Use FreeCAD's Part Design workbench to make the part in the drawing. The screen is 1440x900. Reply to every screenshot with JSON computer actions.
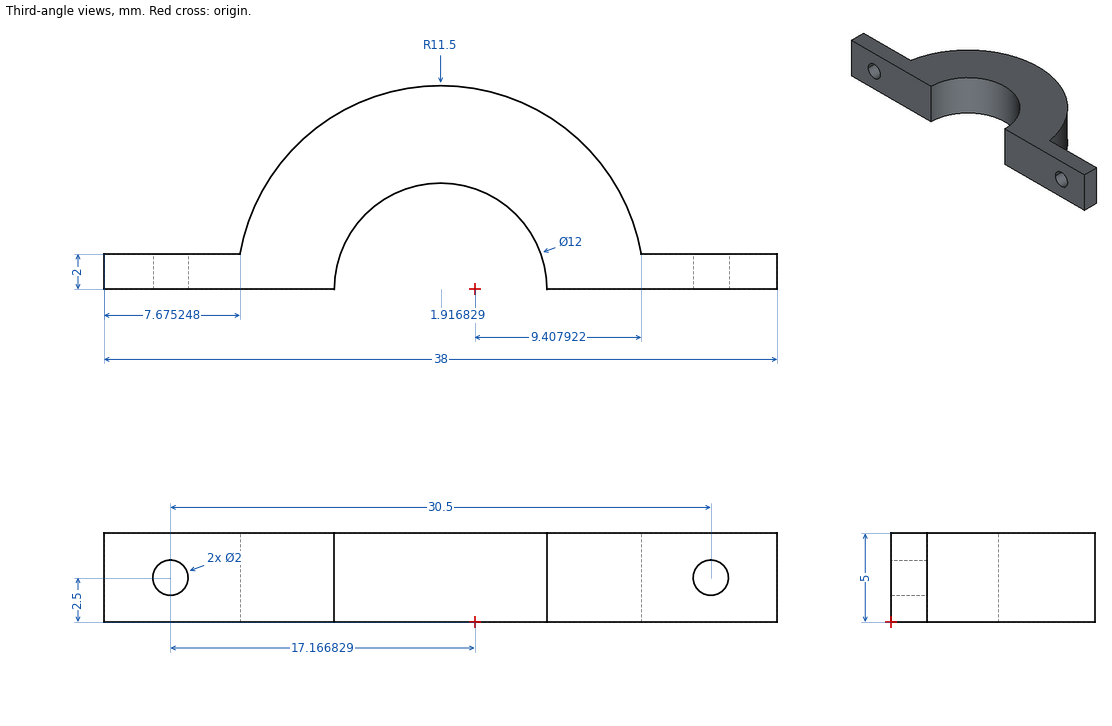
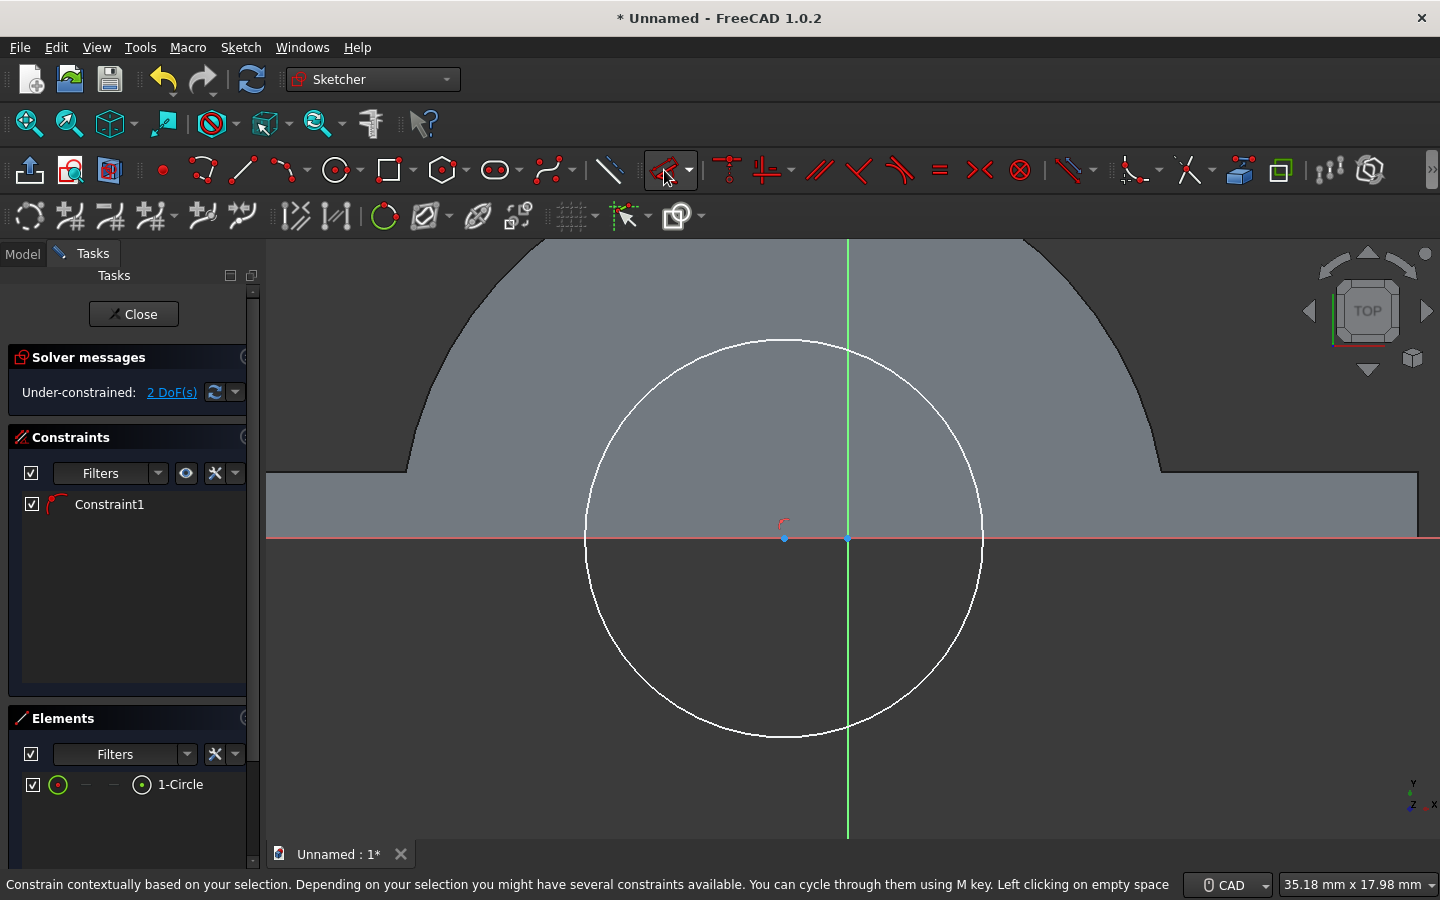
{"action": "left_click", "coordinate": [924, 397]}
{"action": "left_click", "coordinate": [947, 374]}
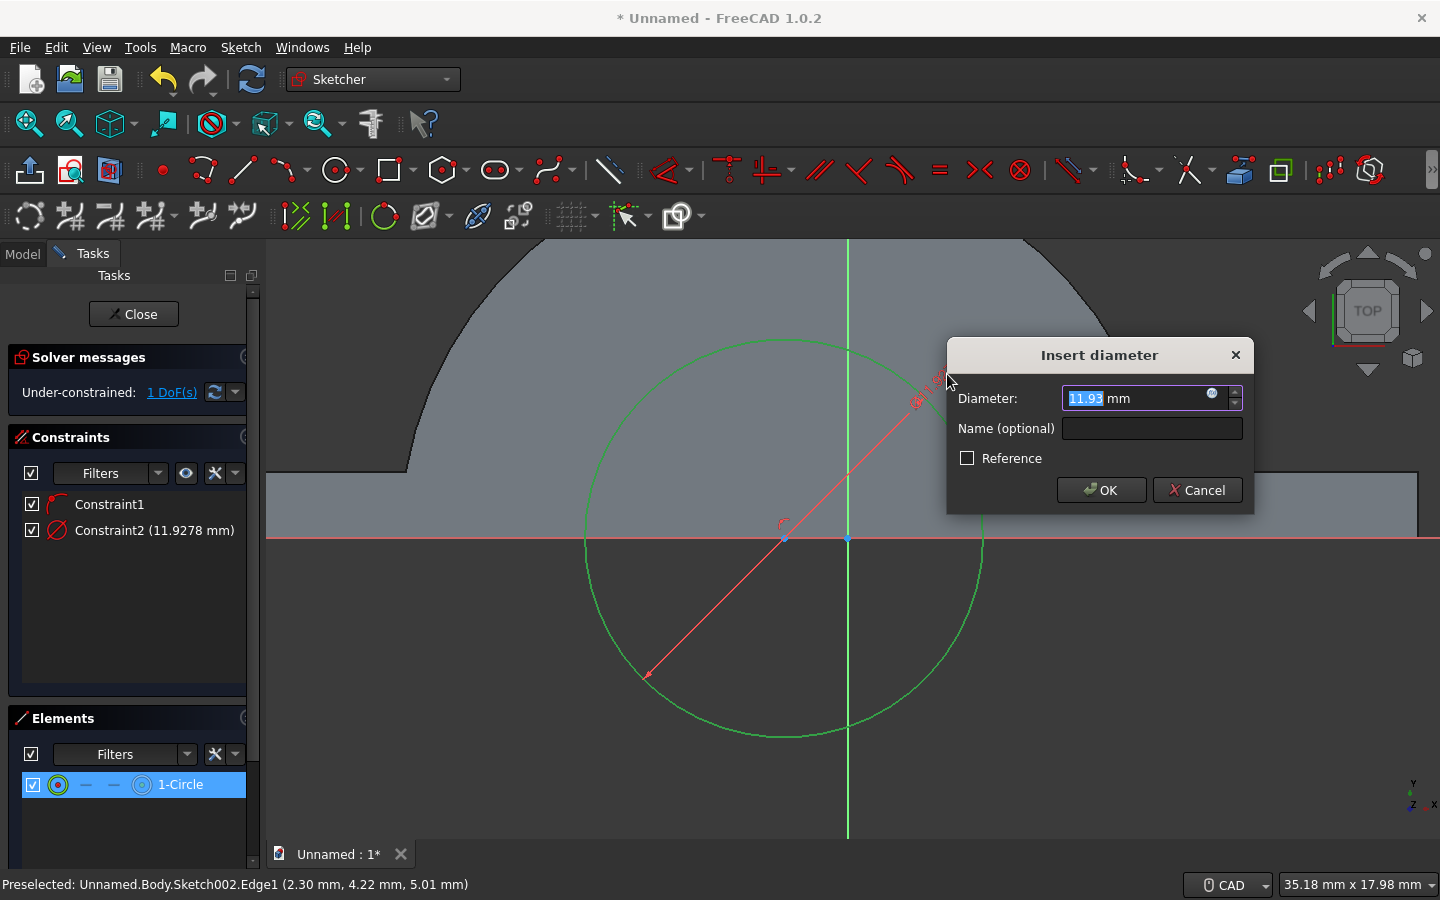
{"action": "type", "text": "12"}
{"action": "key", "text": "Return"}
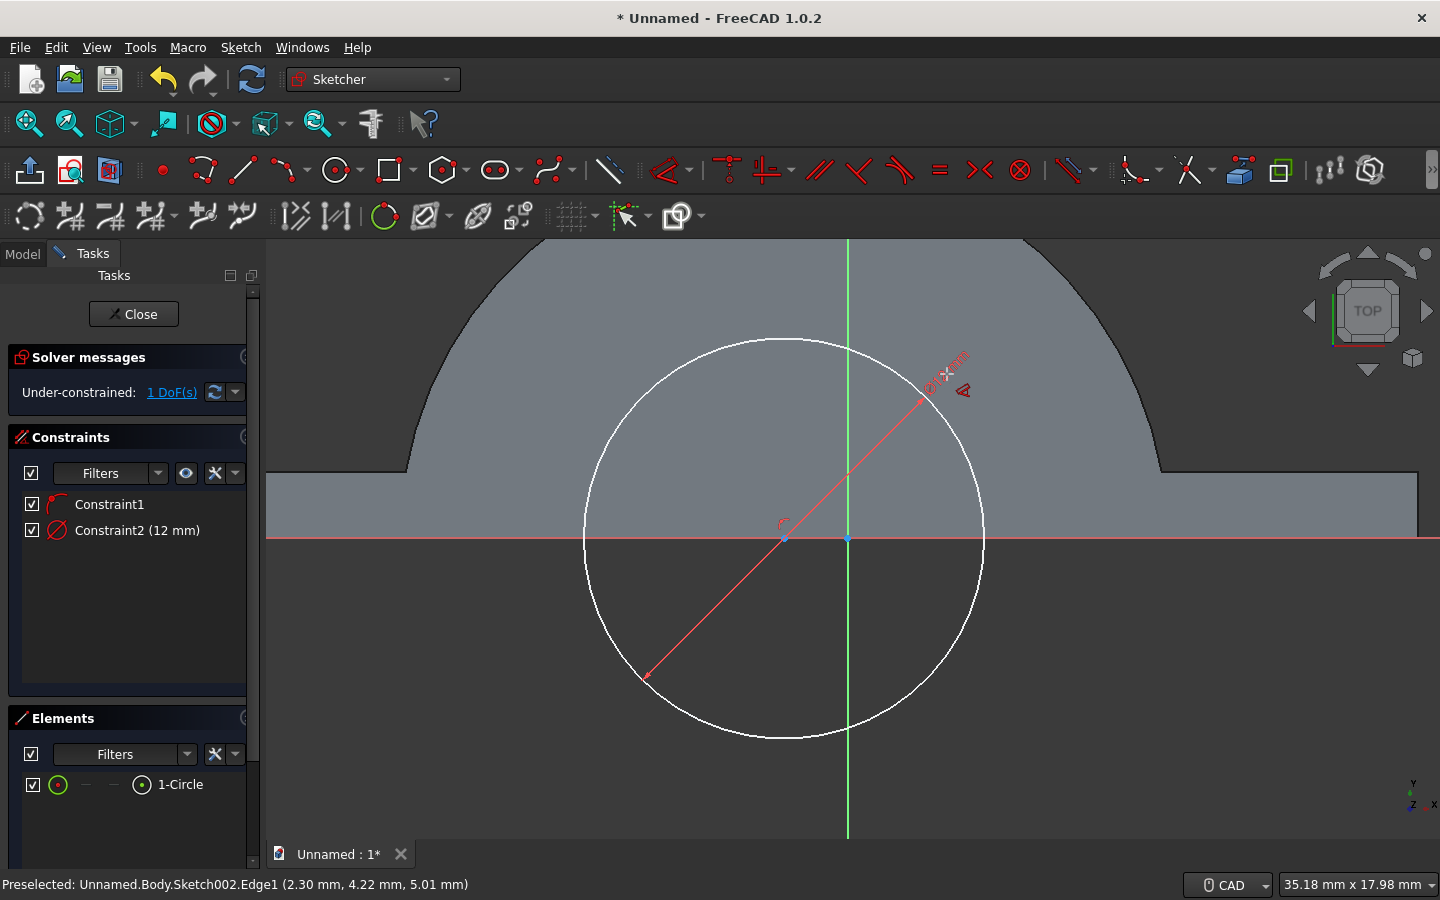
{"action": "left_click", "coordinate": [784, 538]}
{"action": "left_click", "coordinate": [816, 572]}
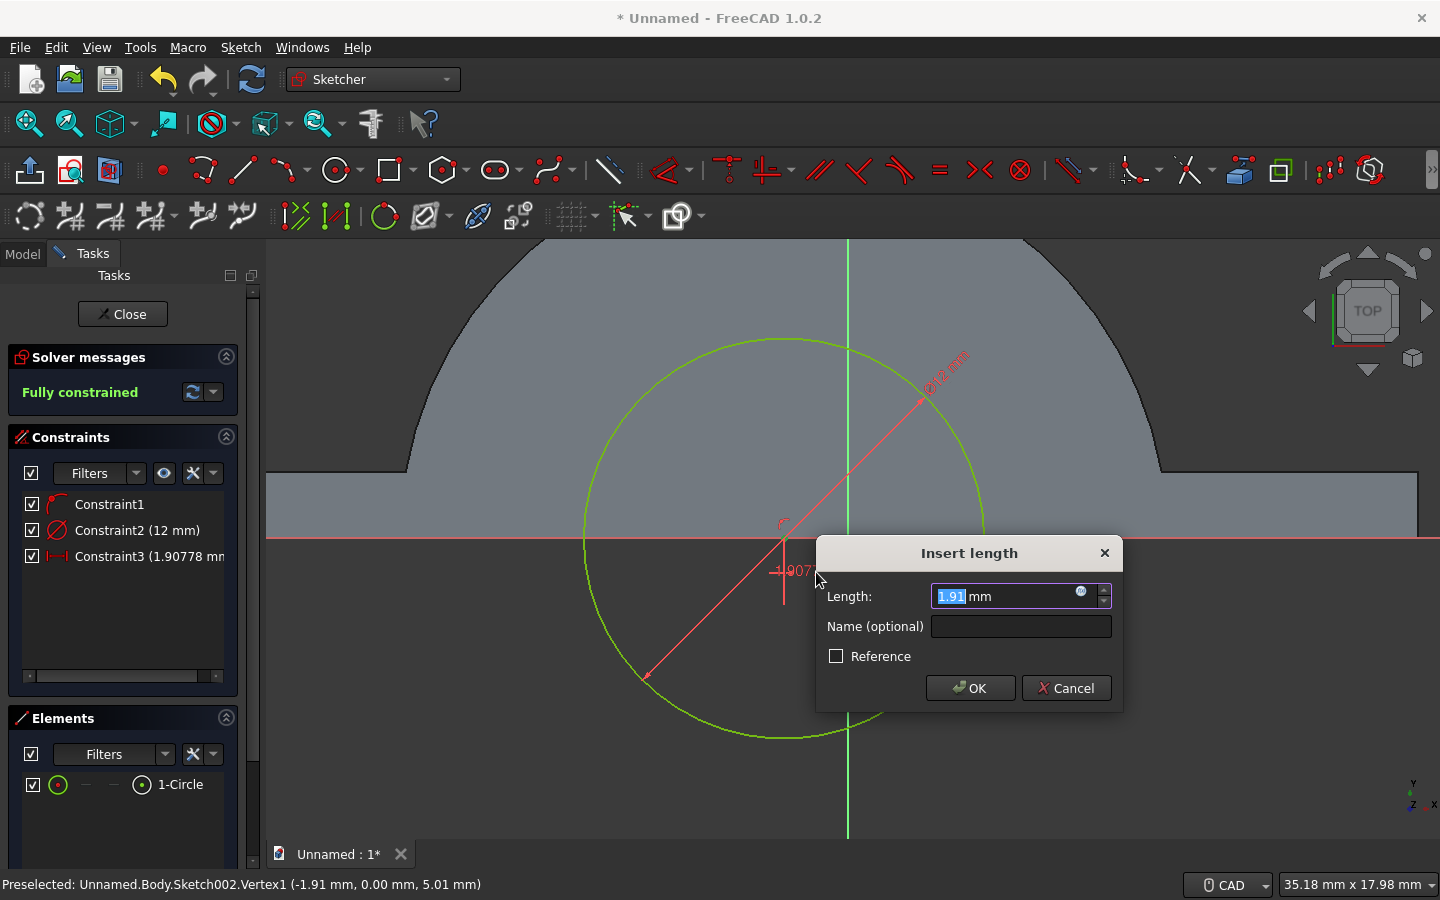
{"action": "type", "text": "1.916829"}
{"action": "key", "text": "Return"}
{"action": "key", "text": "Escape"}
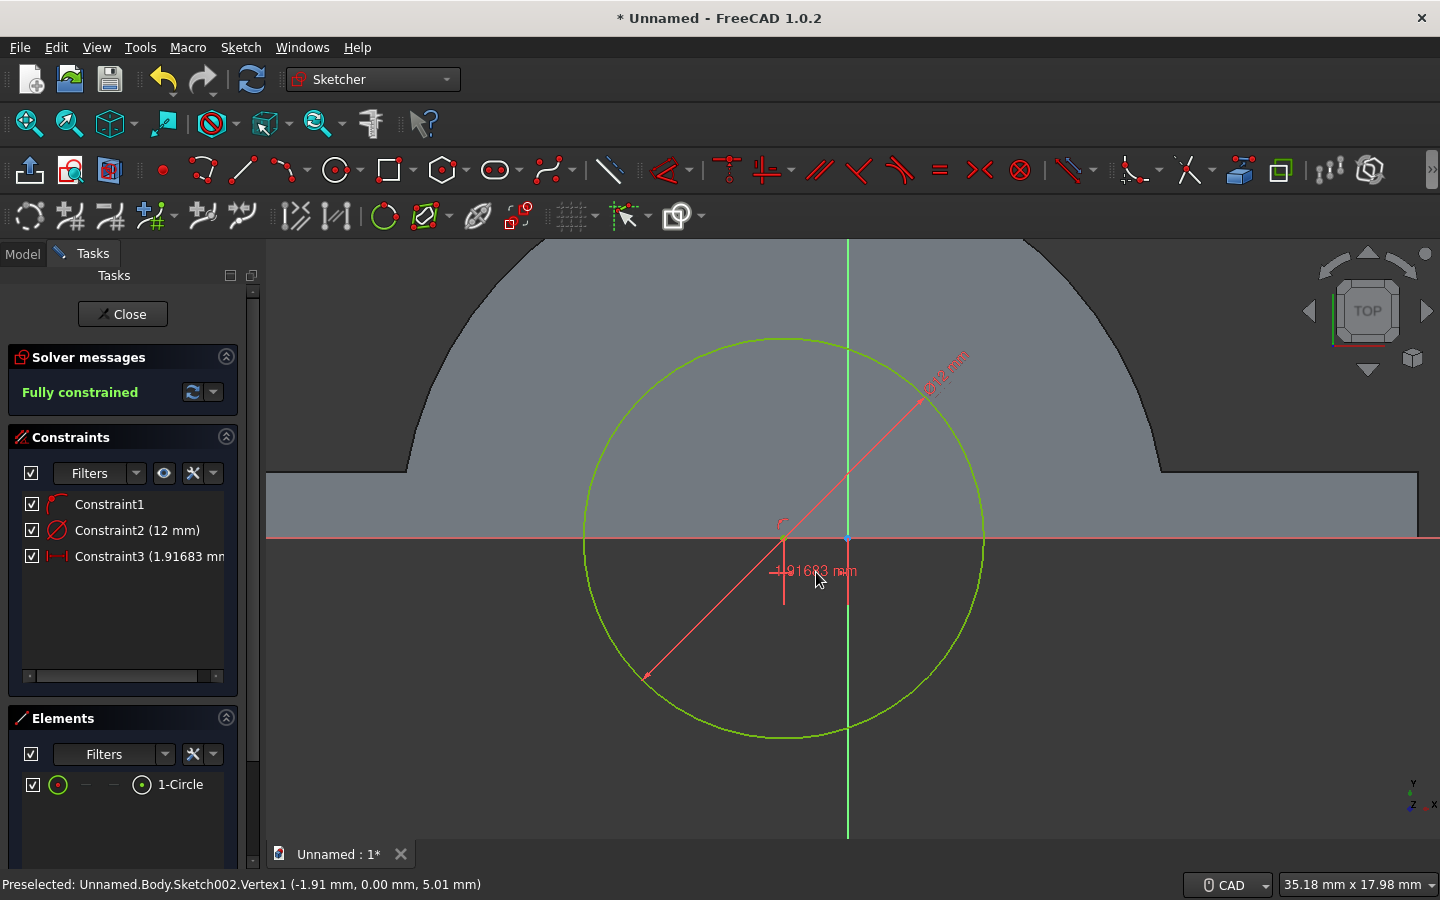
{"action": "left_click", "coordinate": [123, 314]}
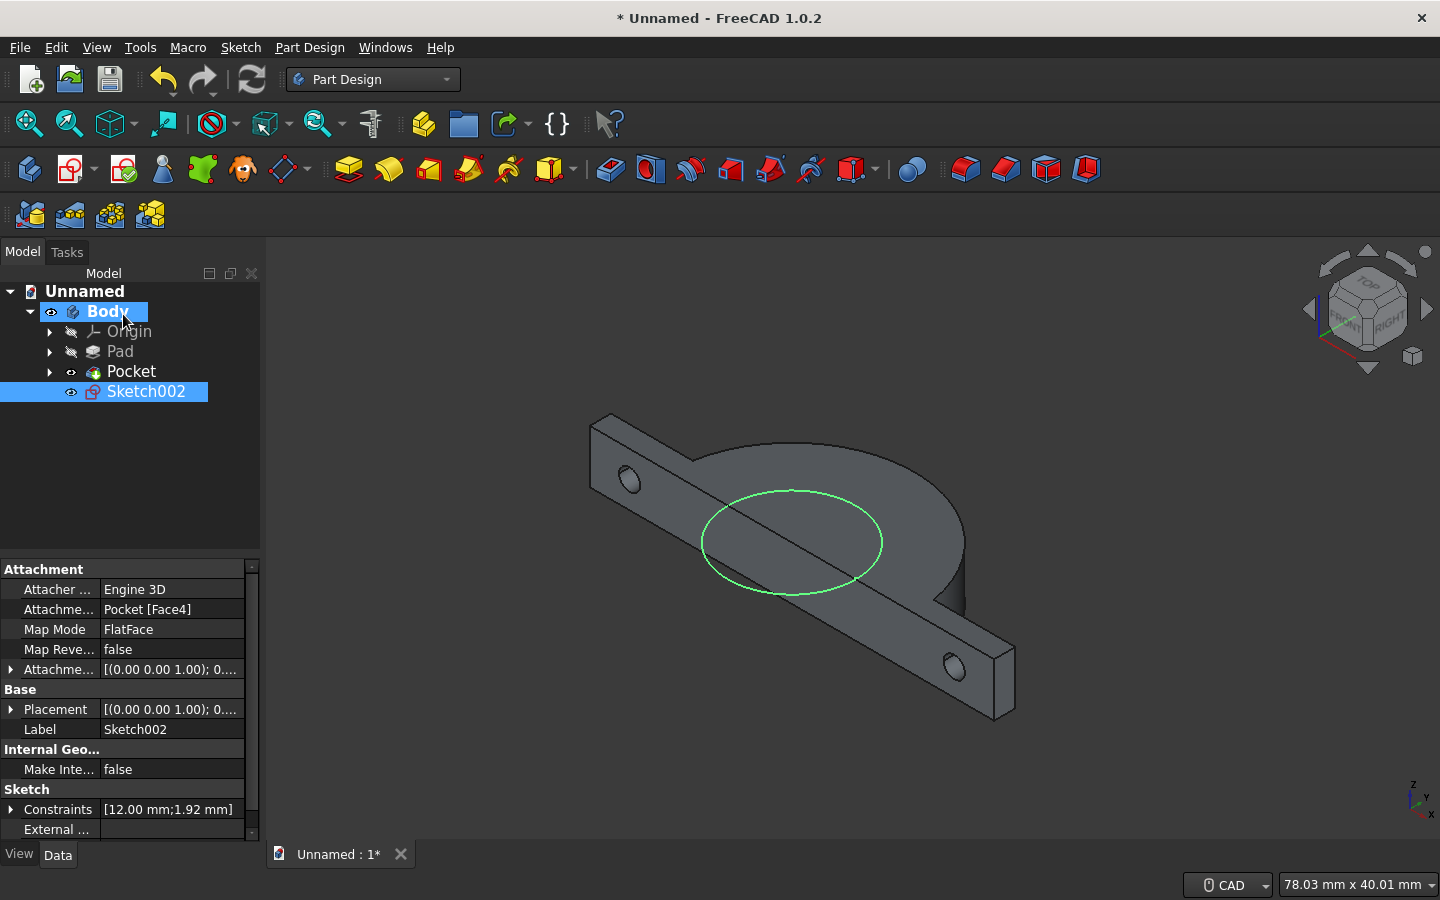
{"action": "left_click", "coordinate": [612, 170]}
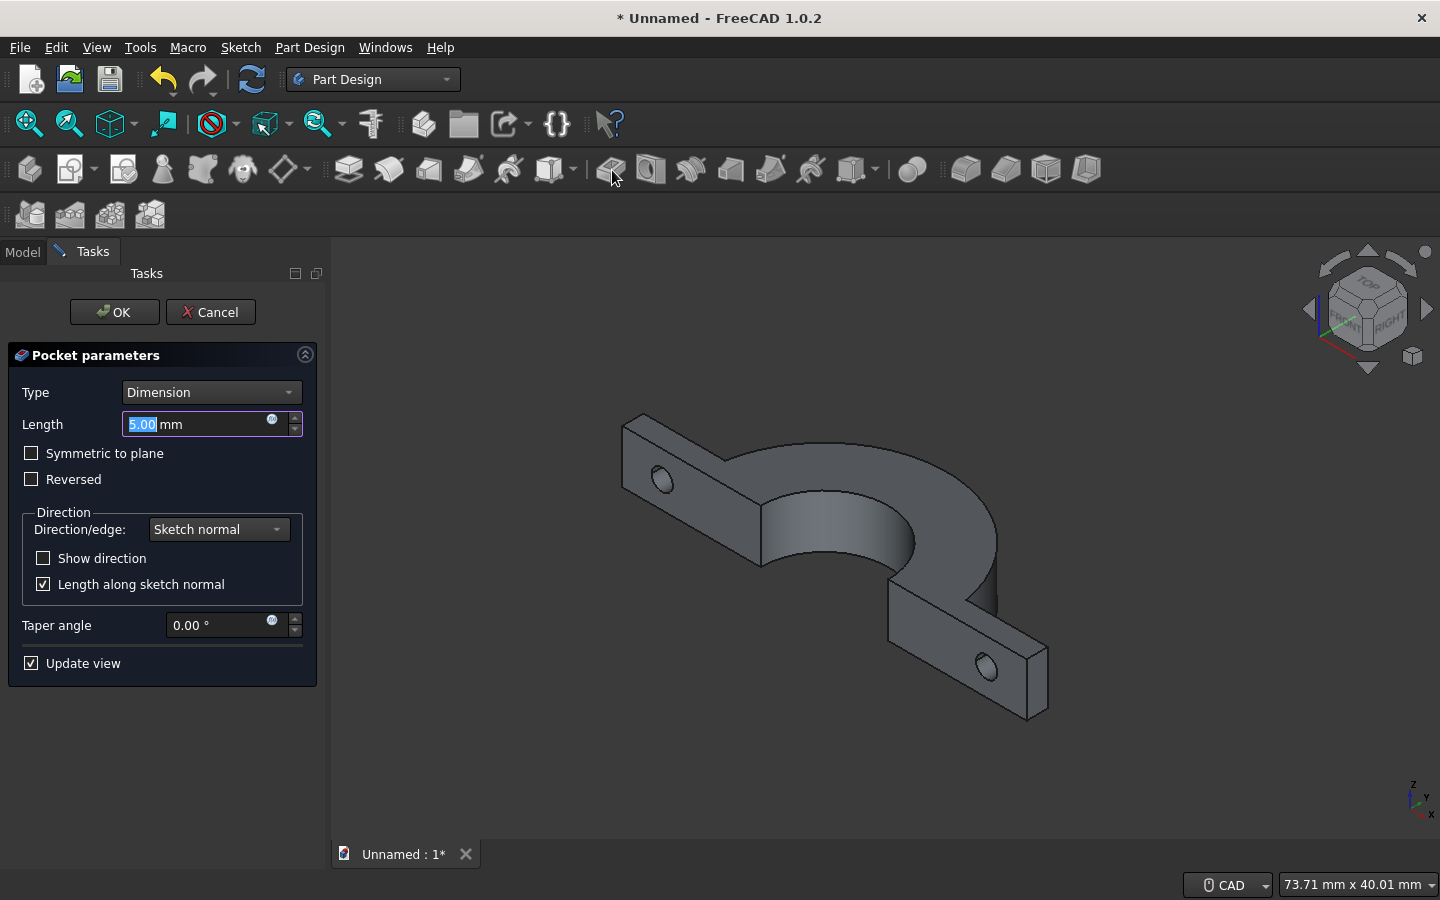
{"action": "left_click", "coordinate": [212, 392]}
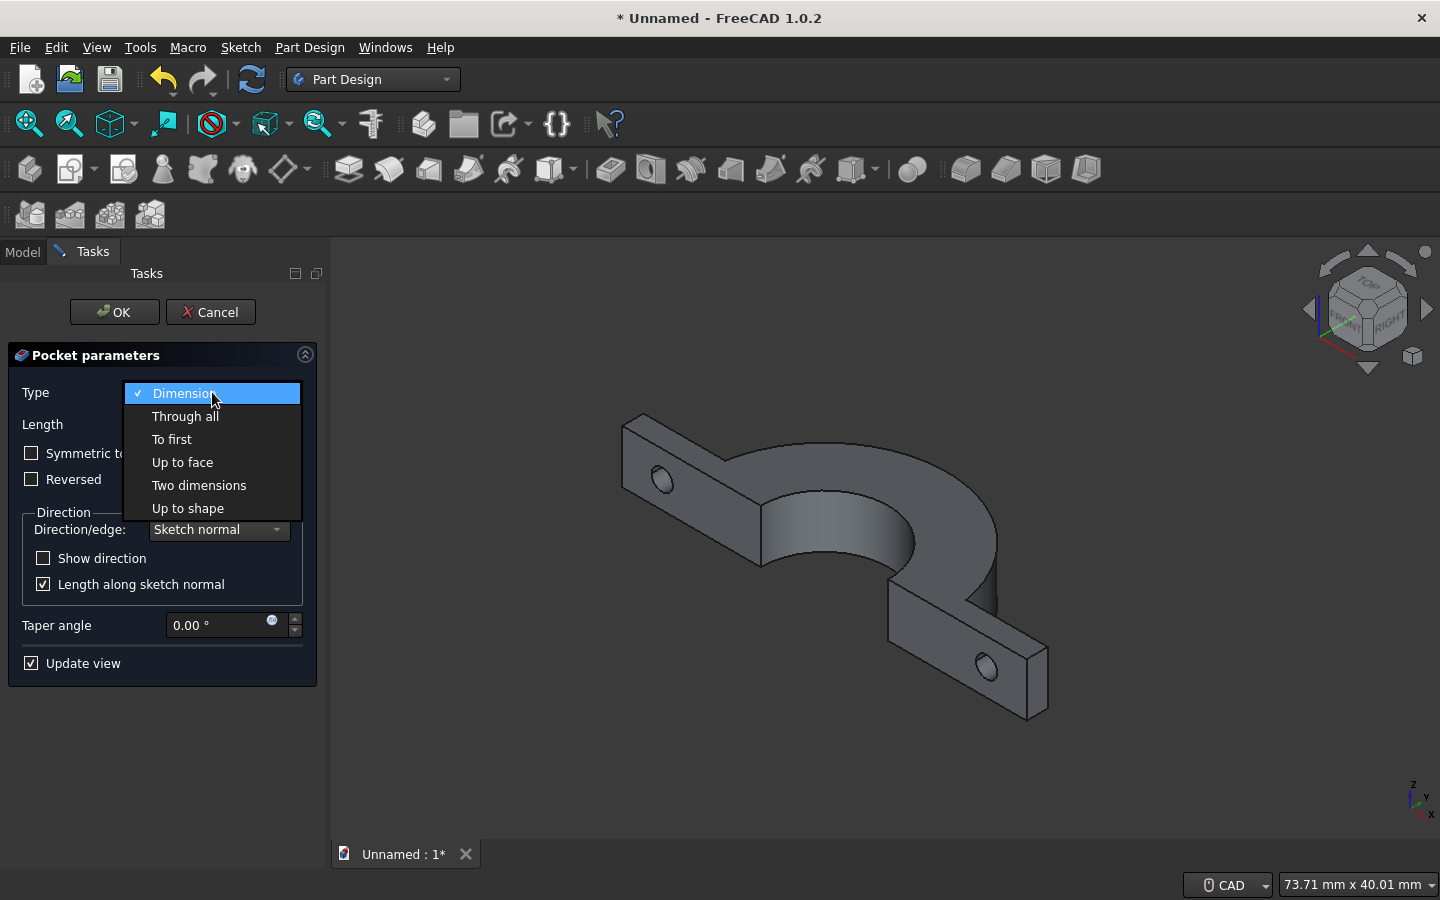
{"action": "left_click", "coordinate": [212, 416]}